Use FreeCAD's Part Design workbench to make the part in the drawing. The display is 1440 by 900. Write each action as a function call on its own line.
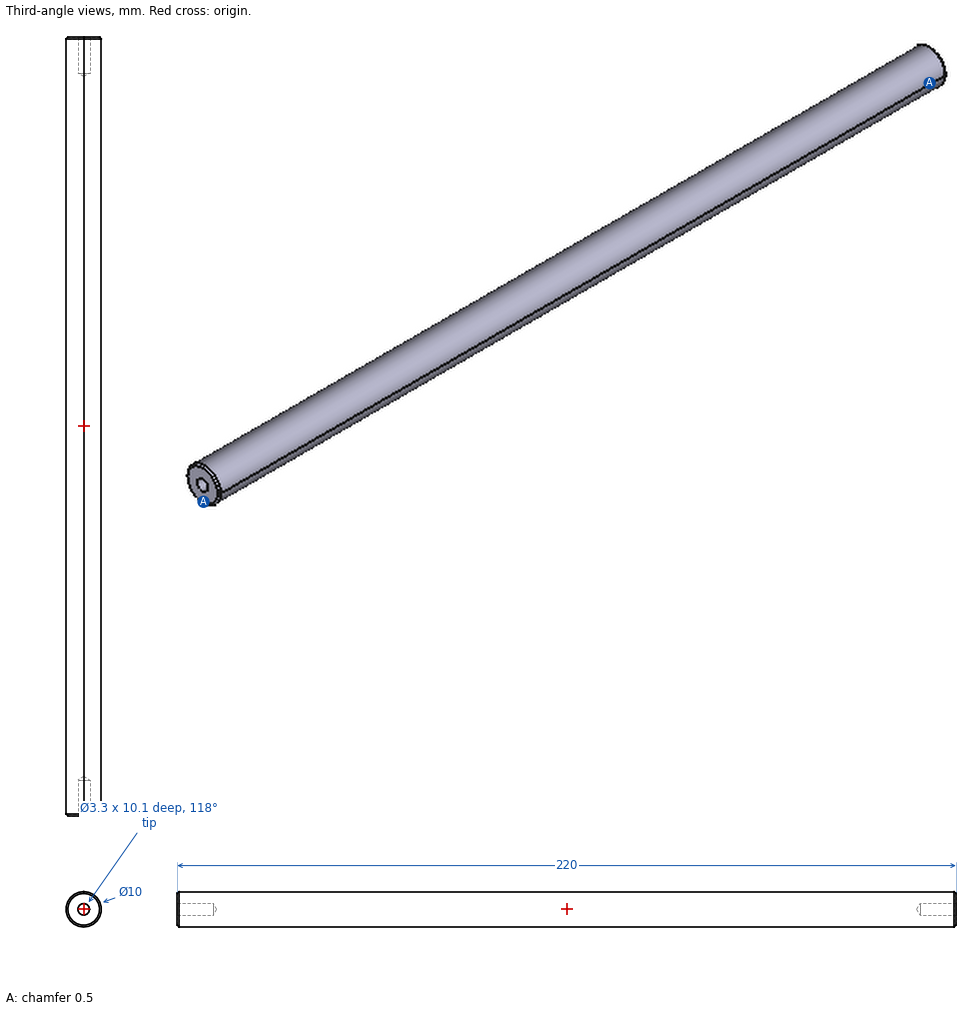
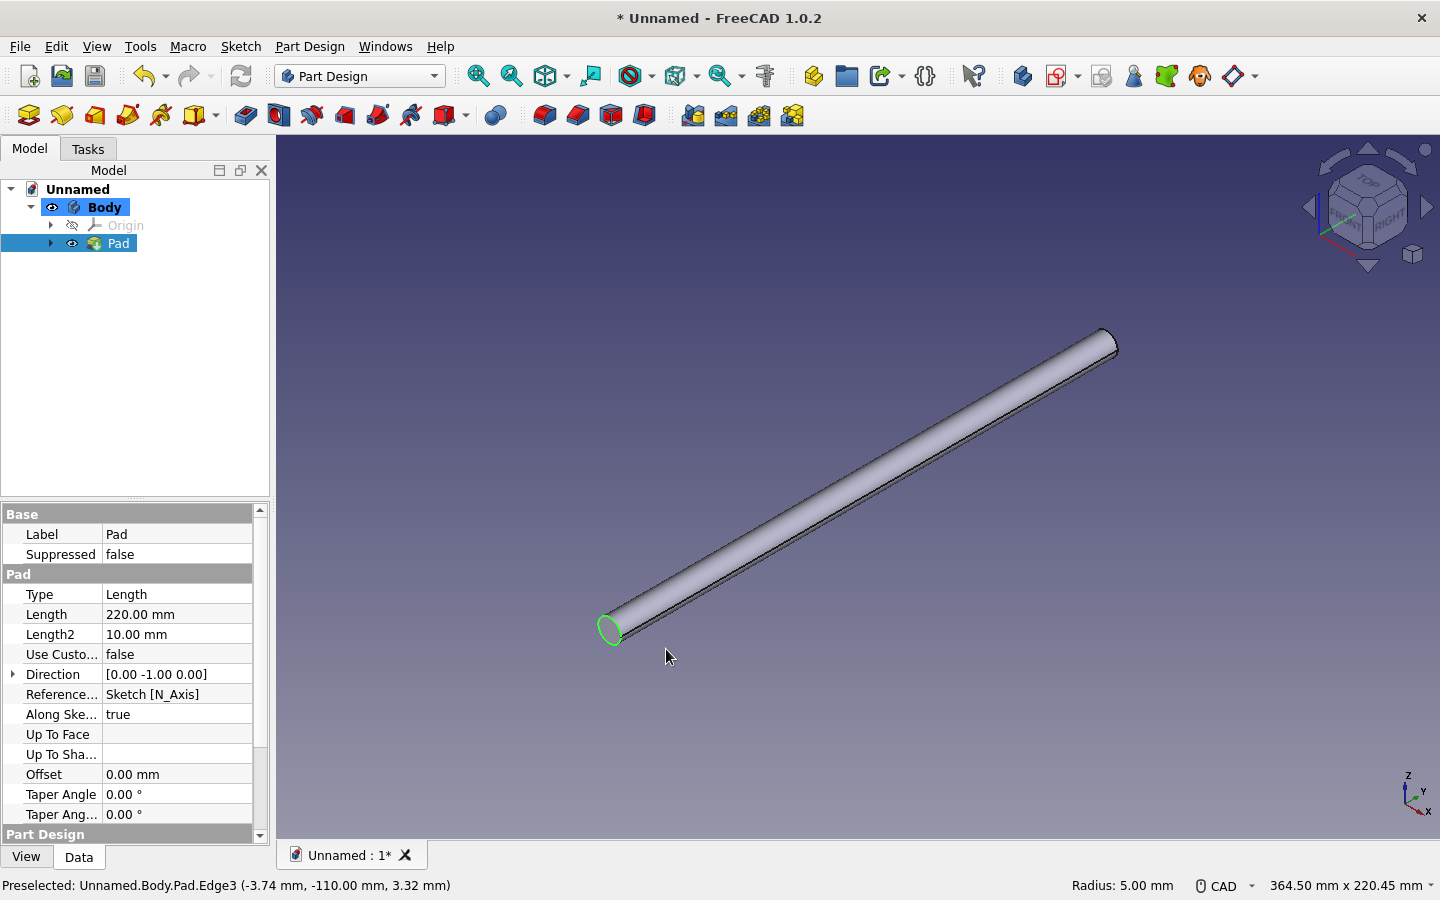
click(1103, 328, ctrl)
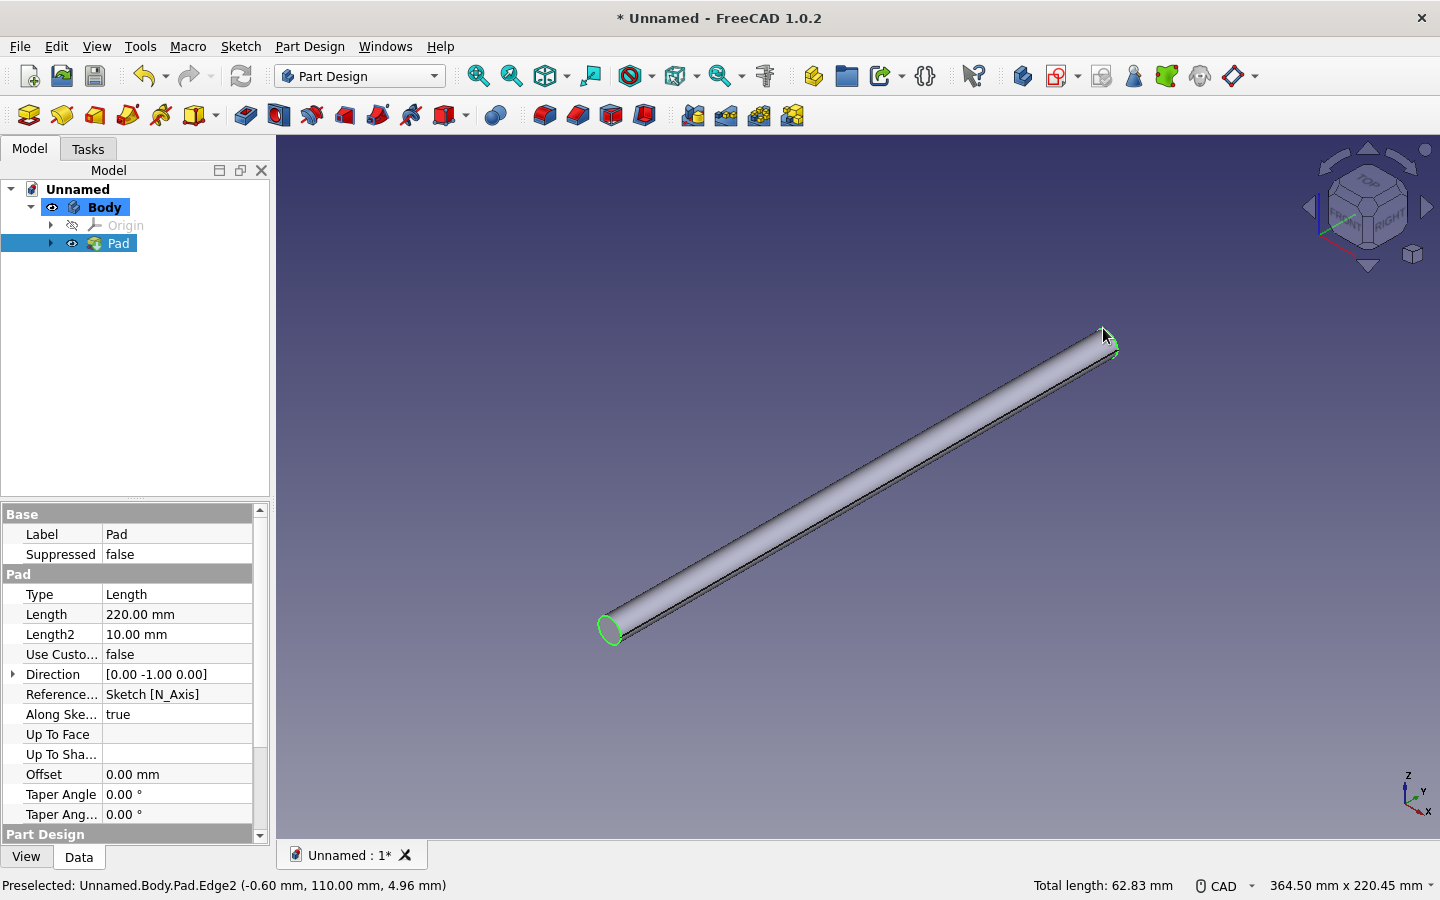
click(578, 116)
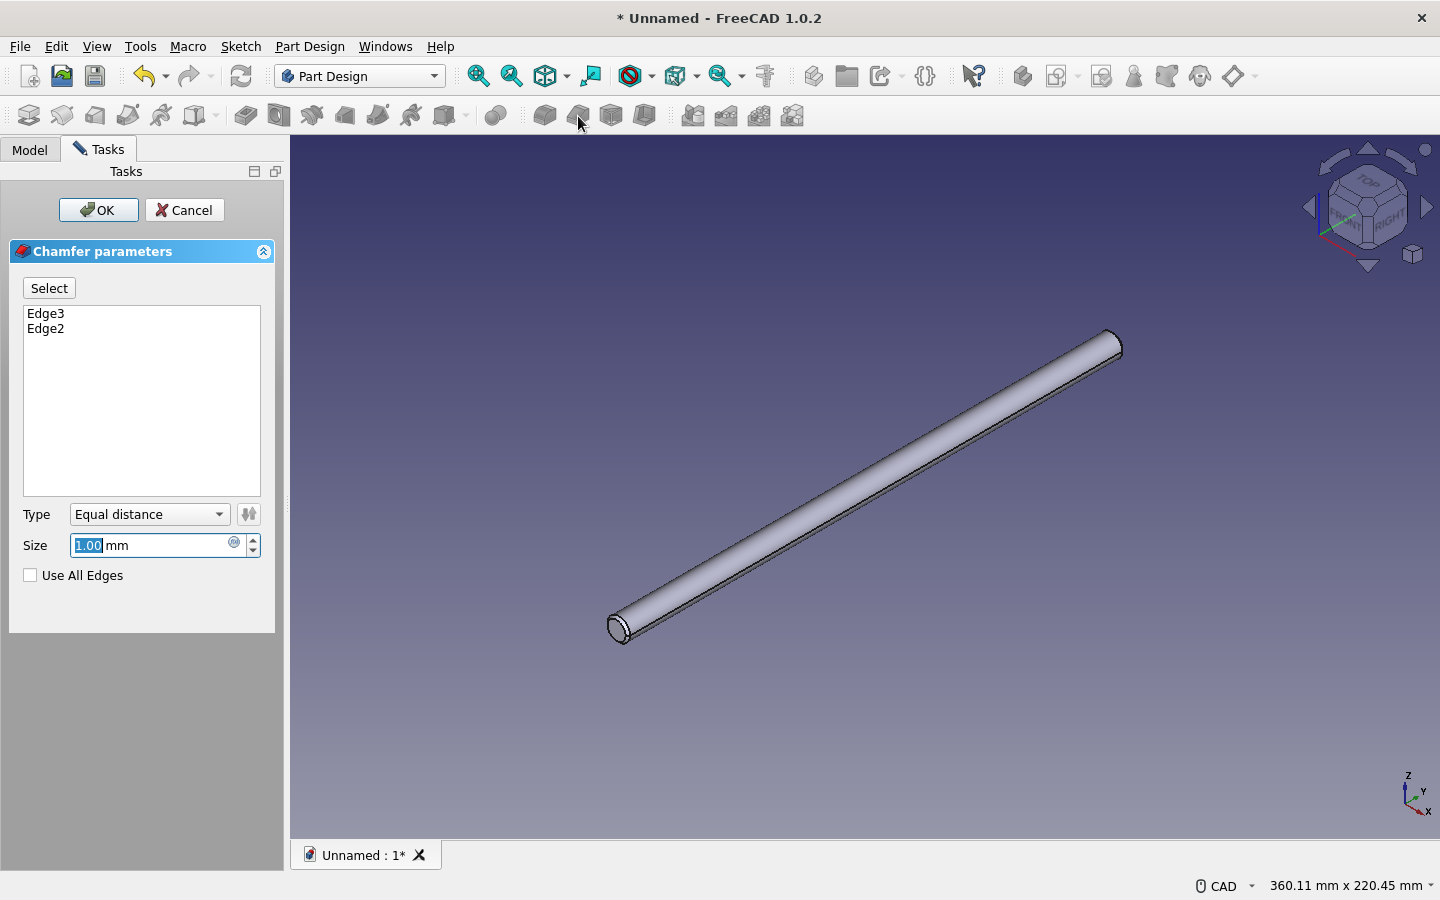
text(0.5)
key(Tab)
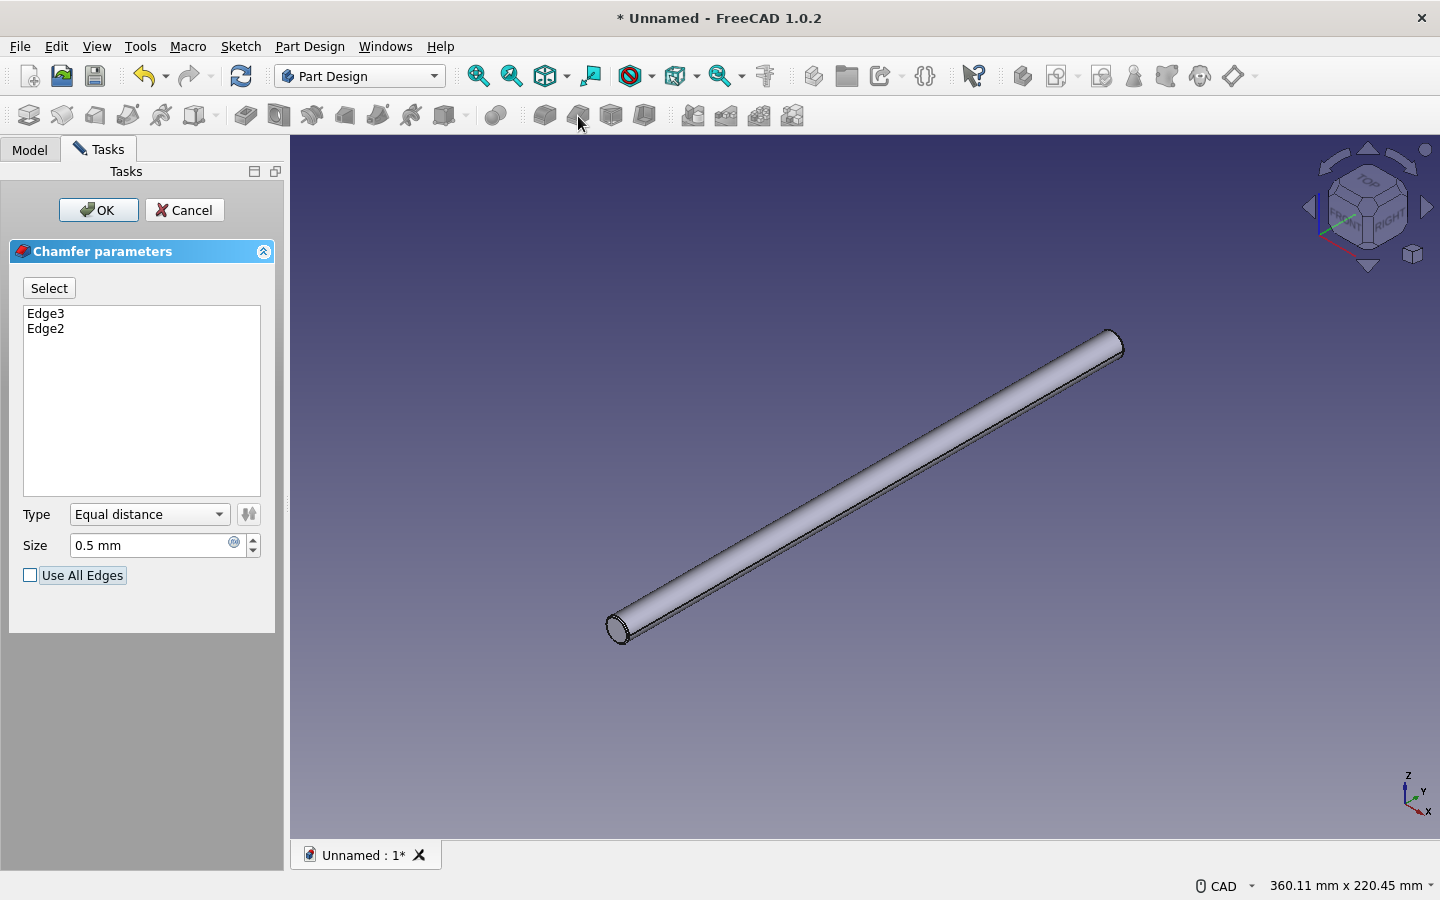
click(99, 210)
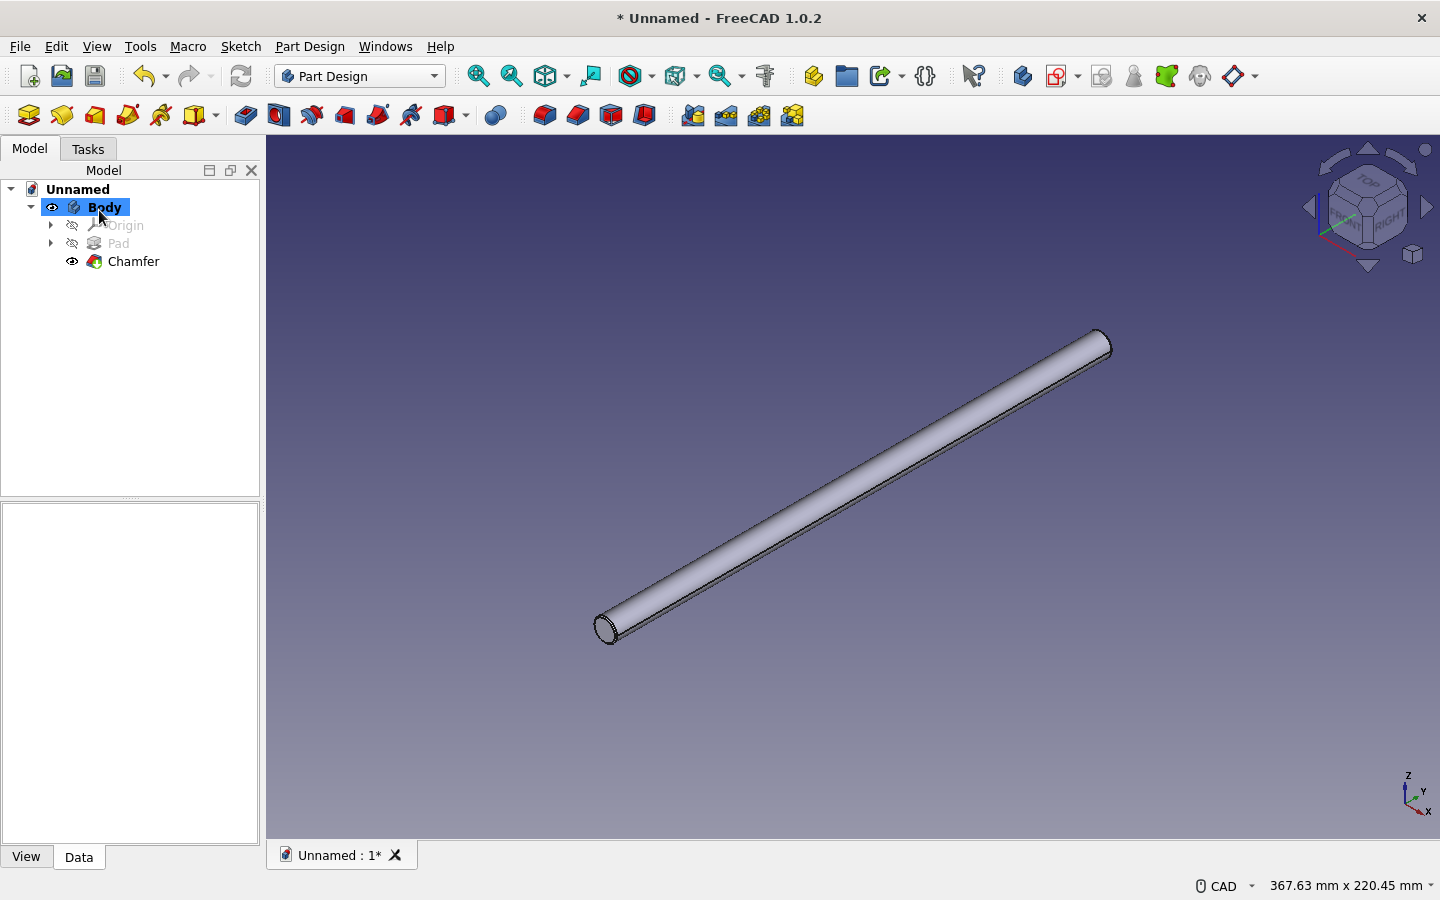
key(4)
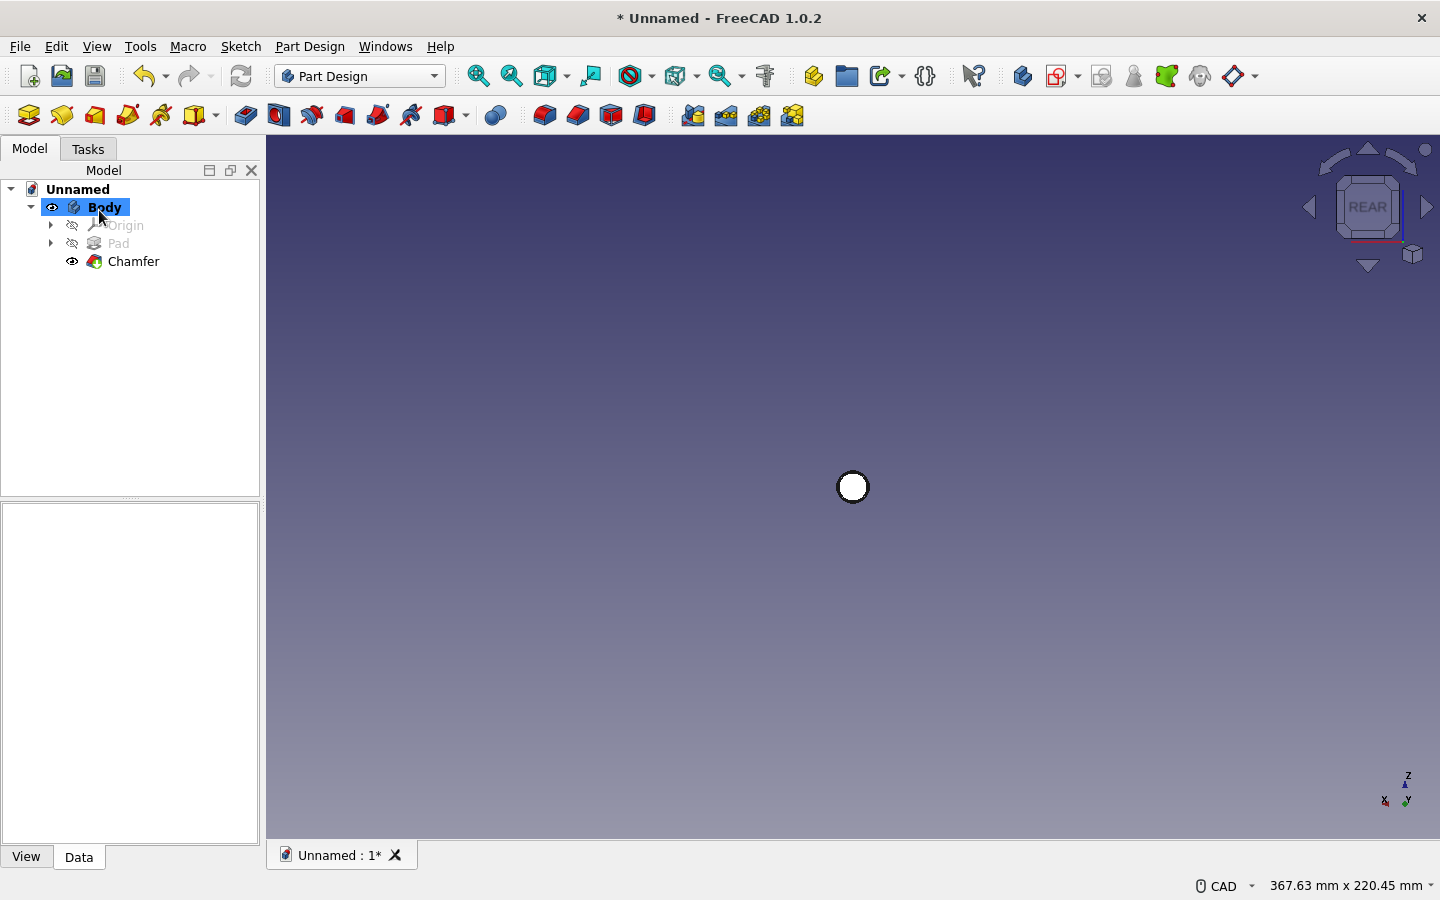
key(v)
key(f)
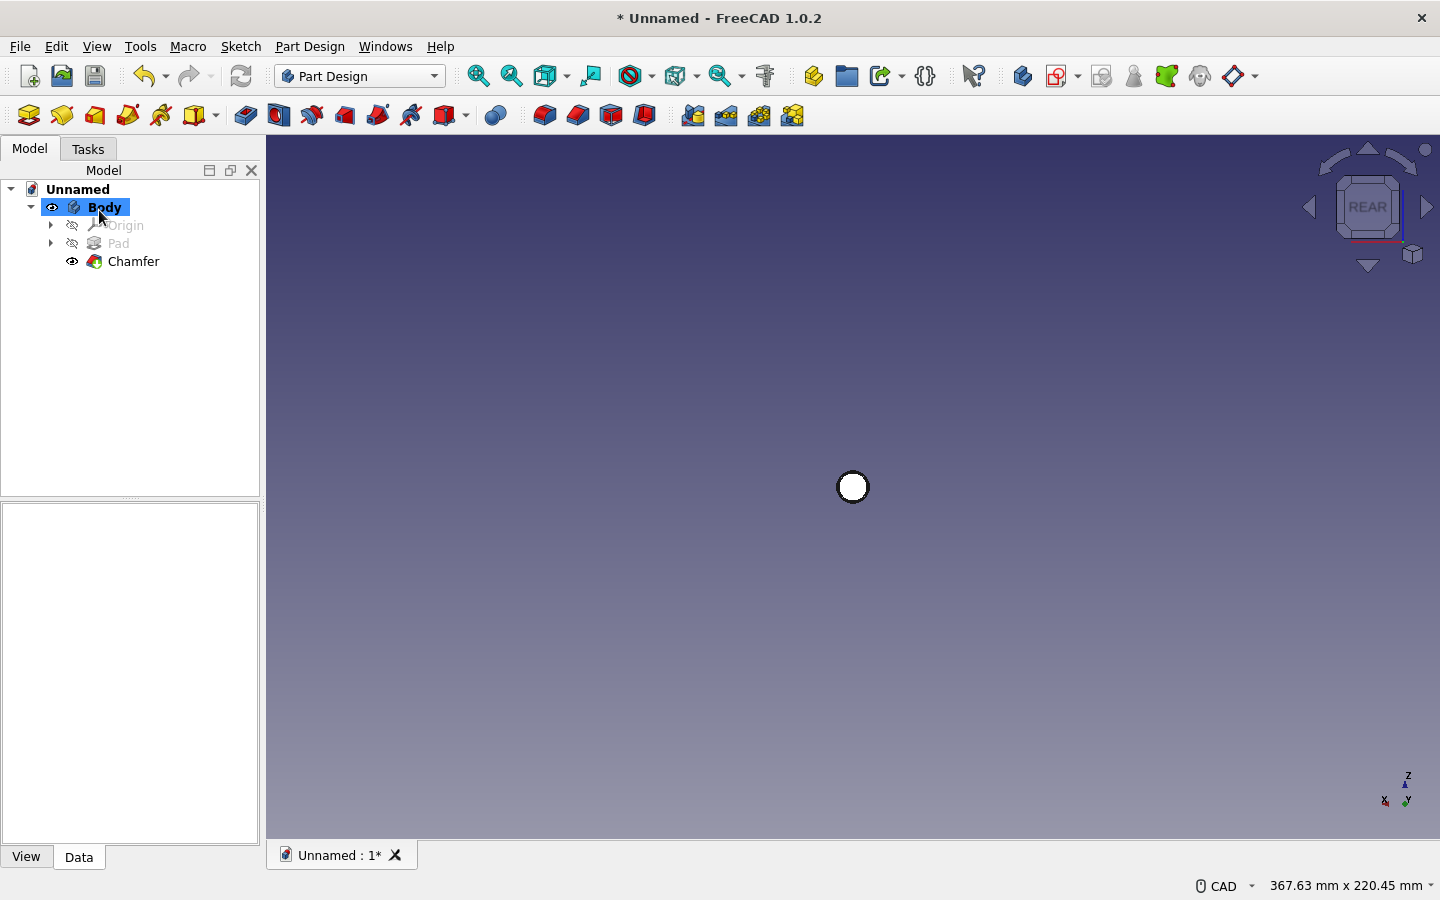
click(853, 486)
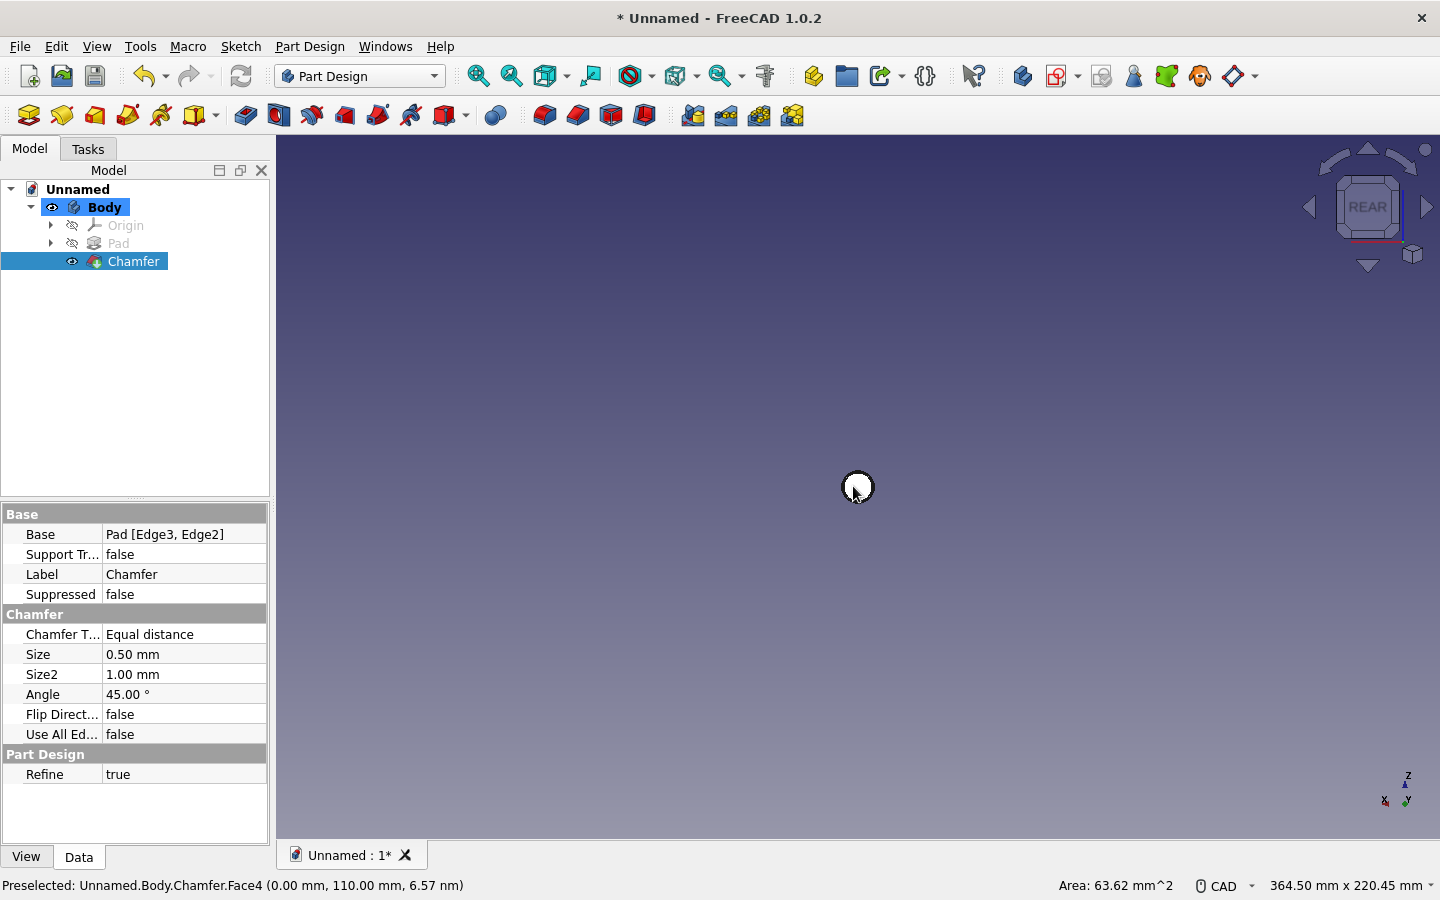
click(1056, 76)